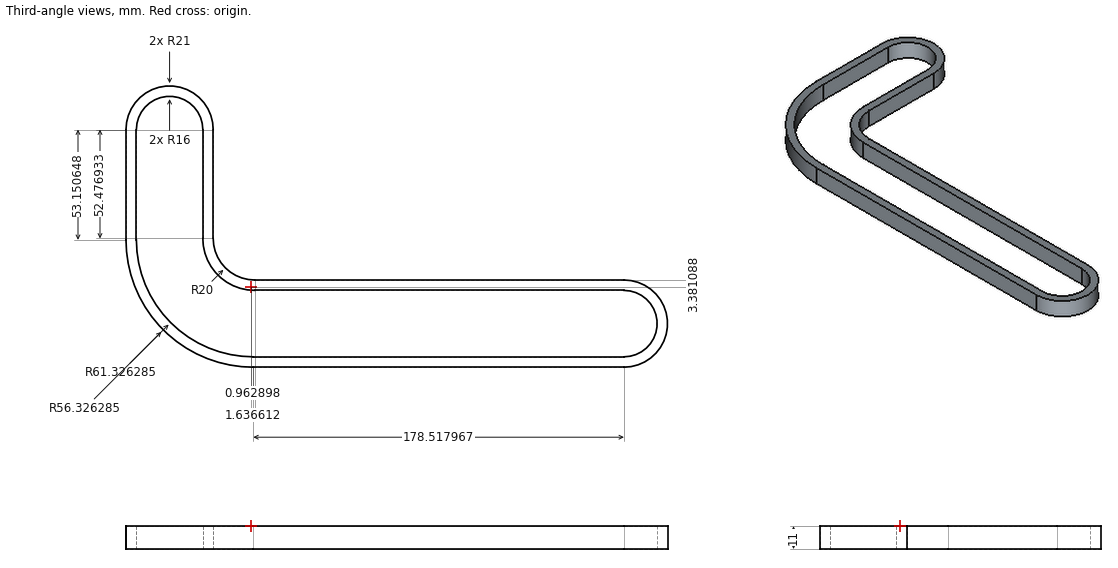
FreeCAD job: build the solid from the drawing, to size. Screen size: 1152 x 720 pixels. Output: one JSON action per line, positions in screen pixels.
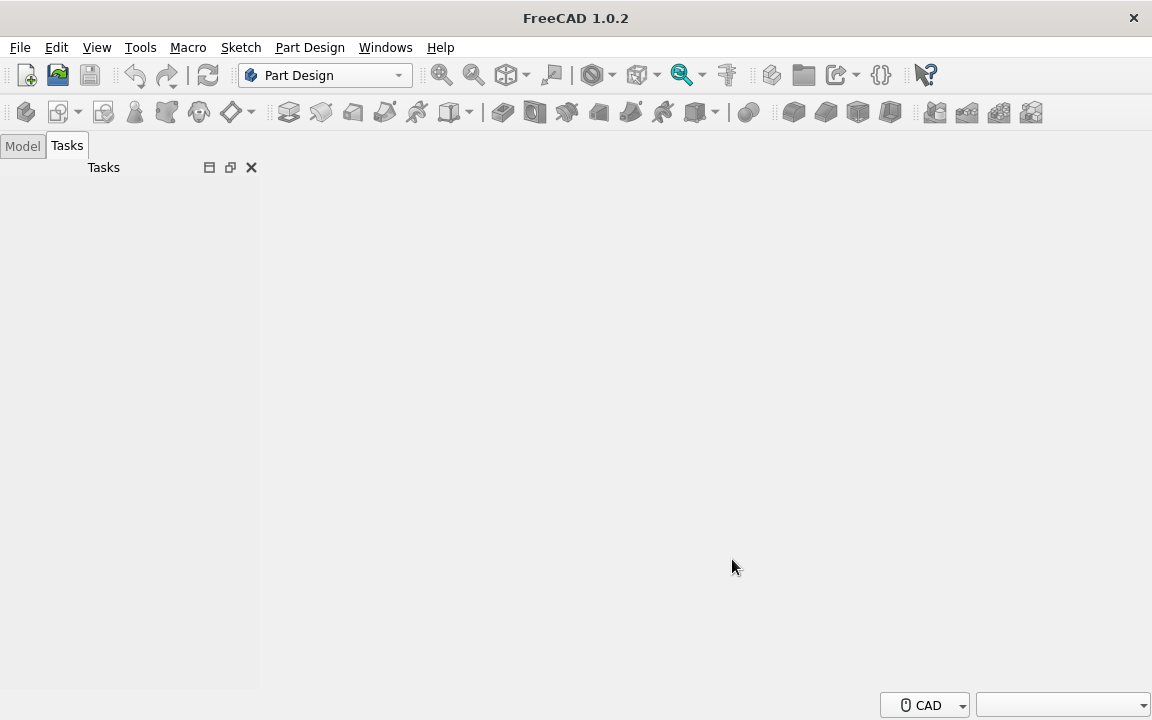
{"action": "key", "text": "ctrl+n"}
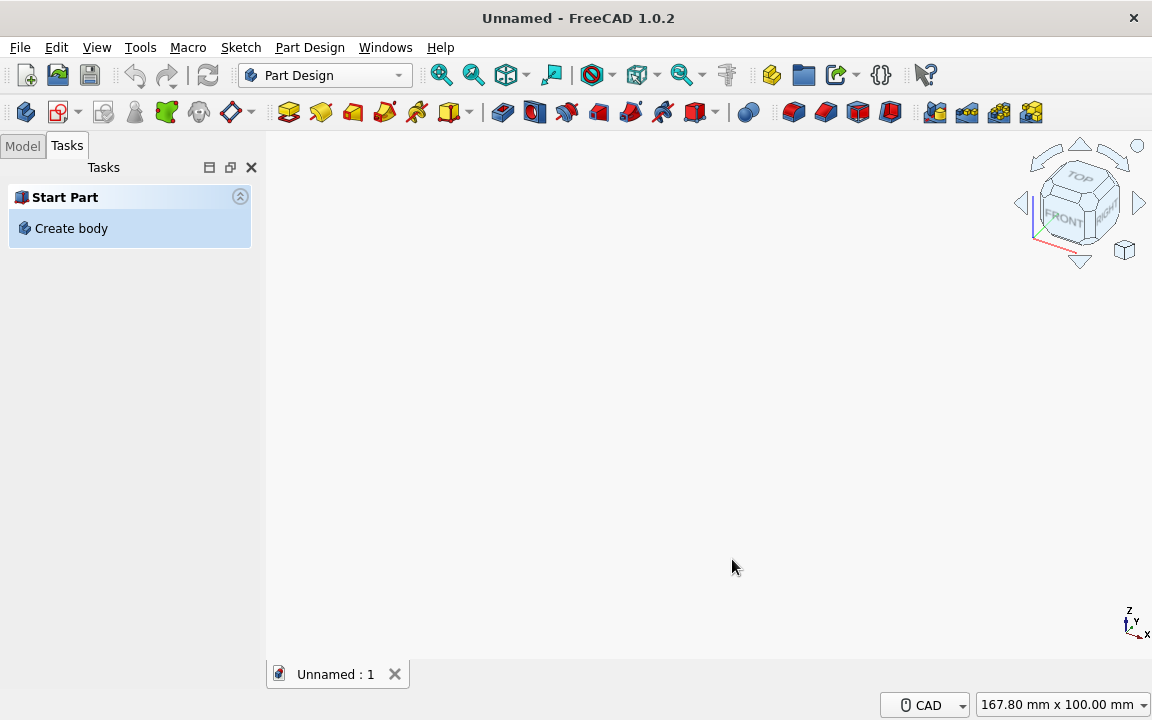
{"action": "left_click", "coordinate": [58, 112]}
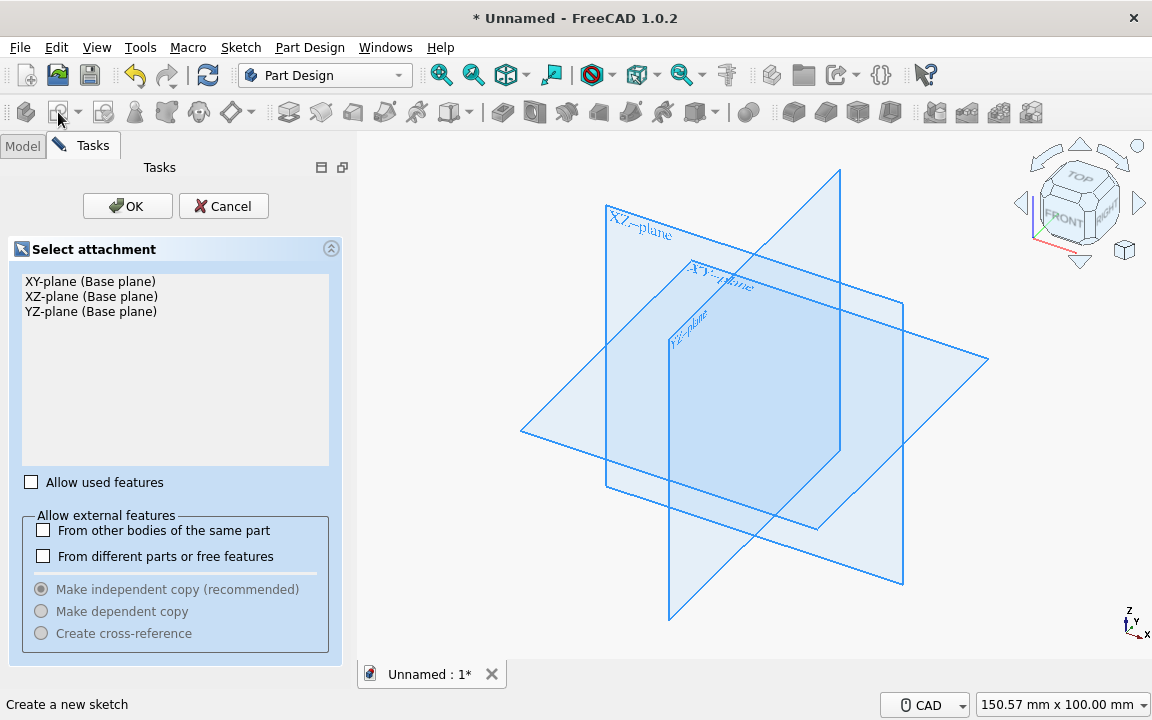
{"action": "left_click", "coordinate": [82, 282]}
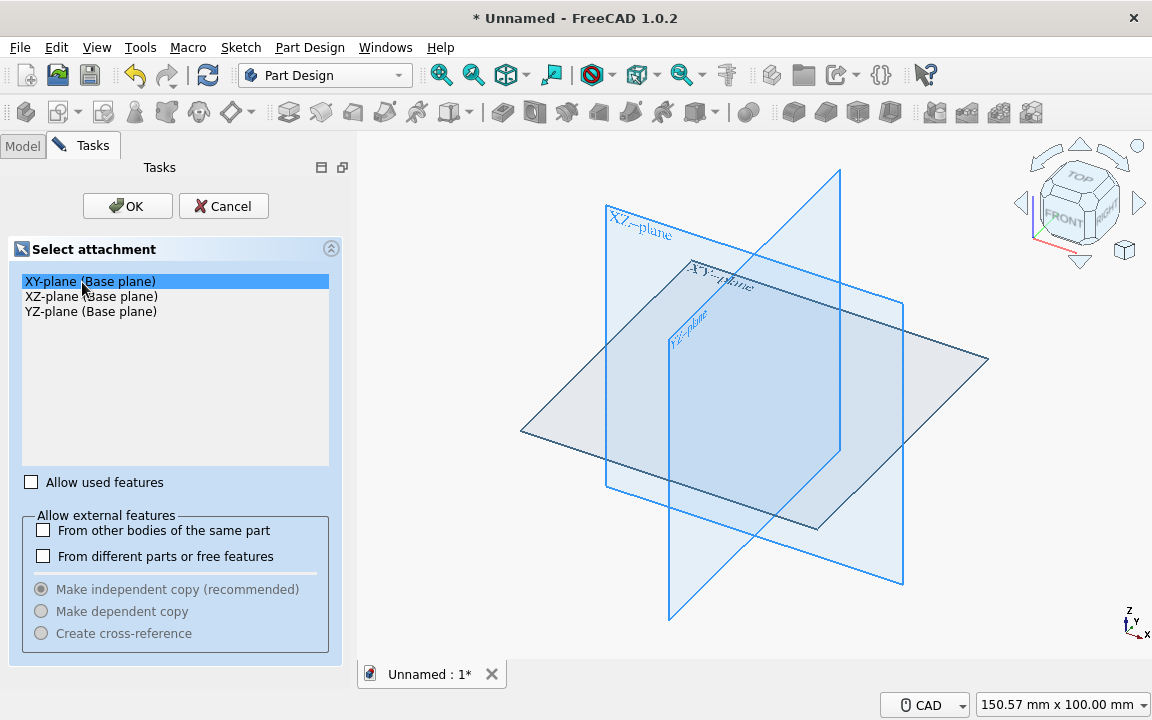
{"action": "left_click", "coordinate": [128, 206]}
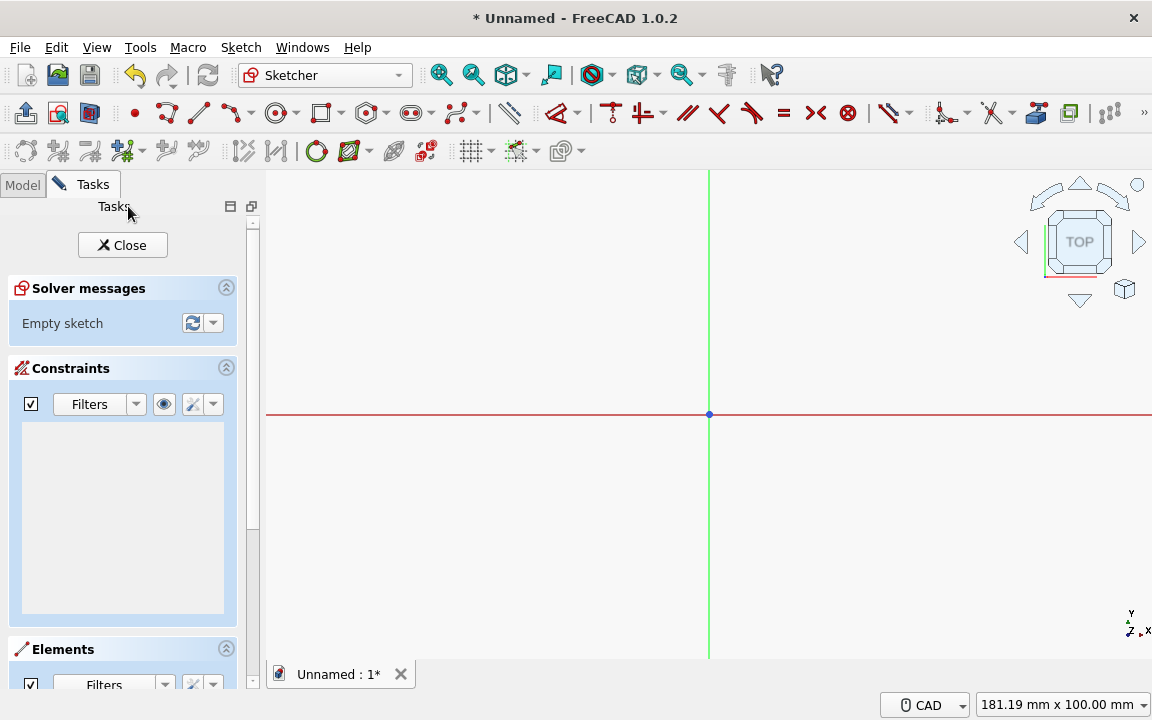
{"action": "scroll", "coordinate": [401, 497], "scroll_direction": "down", "scroll_amount": 5}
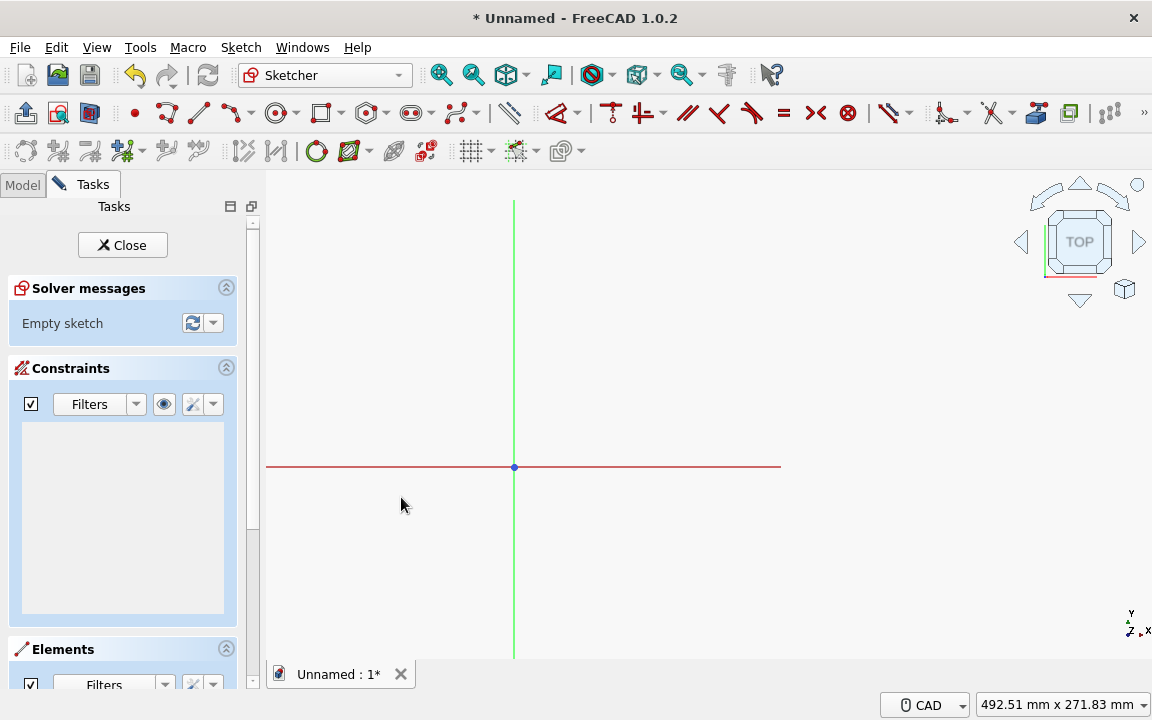
{"action": "left_click", "coordinate": [200, 114]}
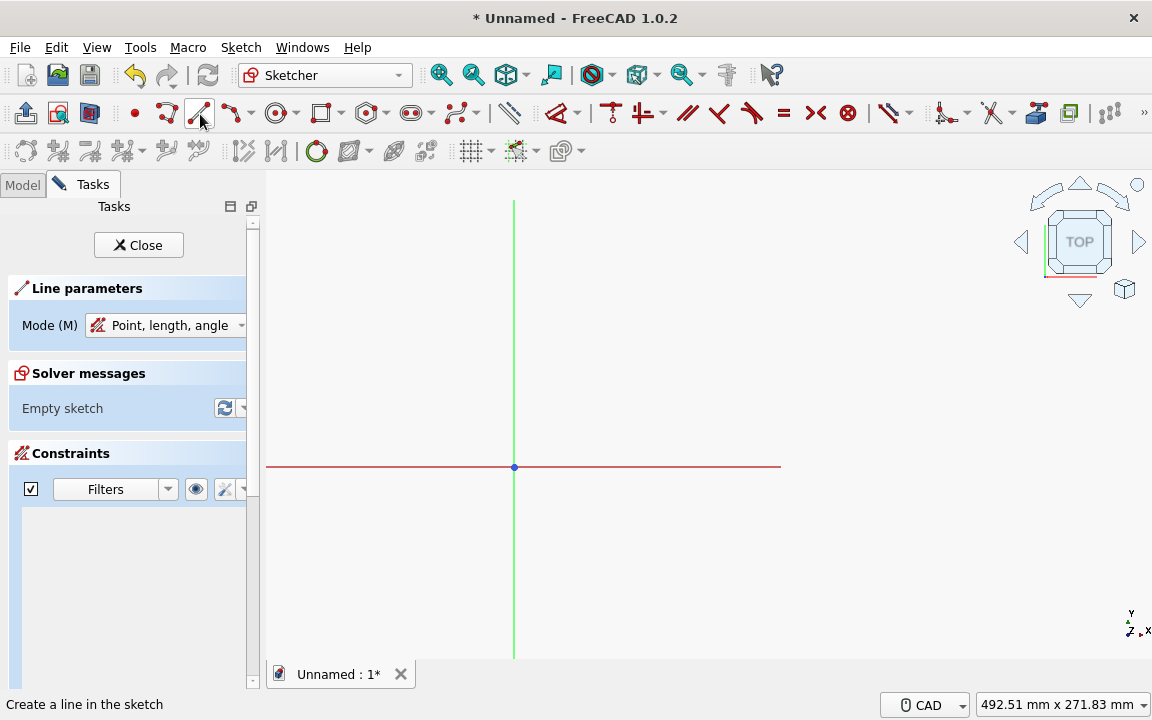
{"action": "left_click", "coordinate": [481, 425]}
{"action": "left_click", "coordinate": [481, 331]}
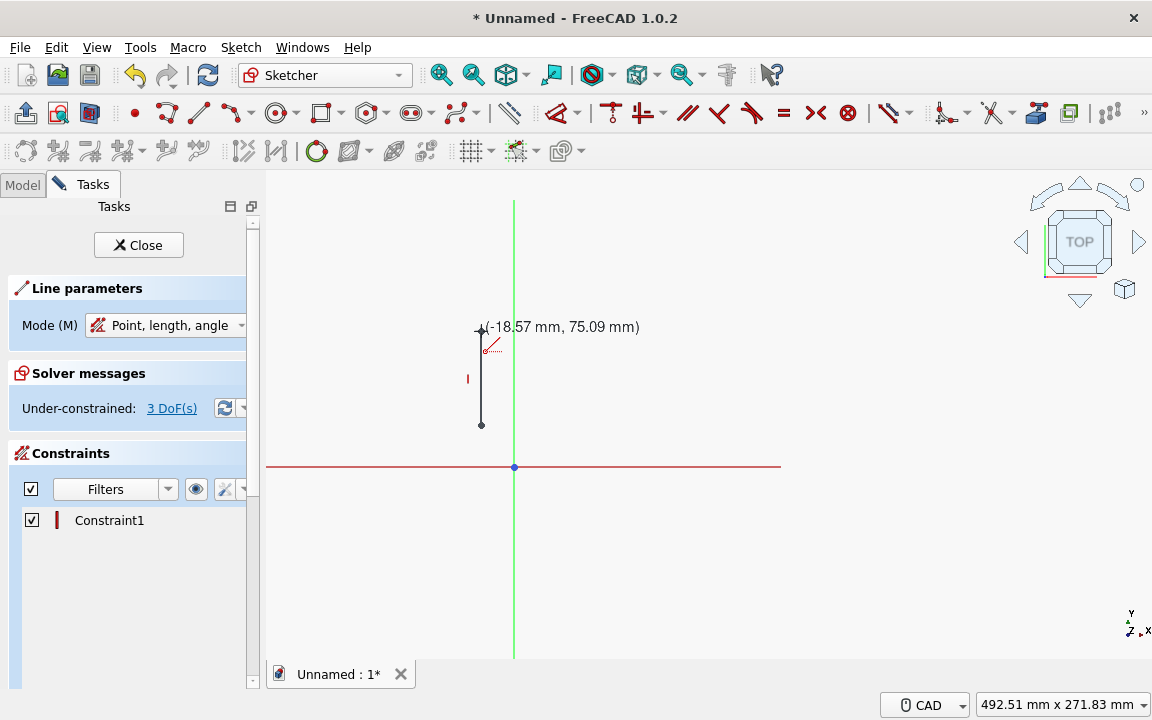
{"action": "left_click", "coordinate": [406, 331]}
{"action": "left_click", "coordinate": [406, 426]}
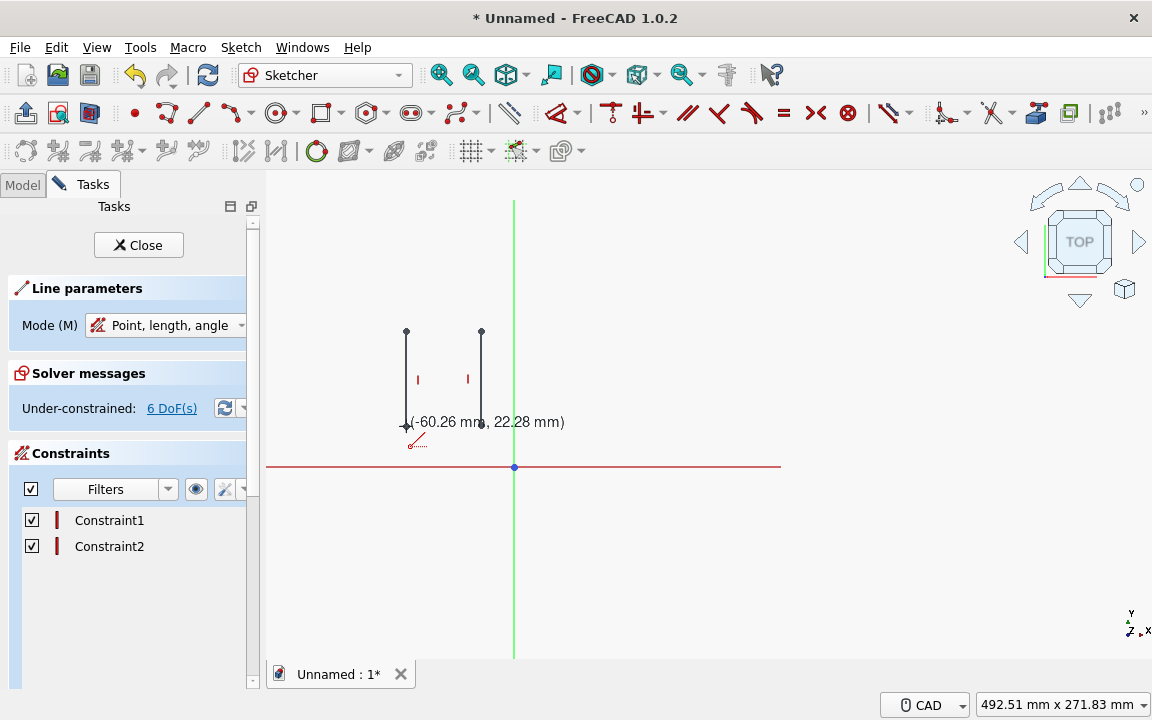
{"action": "scroll", "coordinate": [516, 537], "scroll_direction": "up", "scroll_amount": 12}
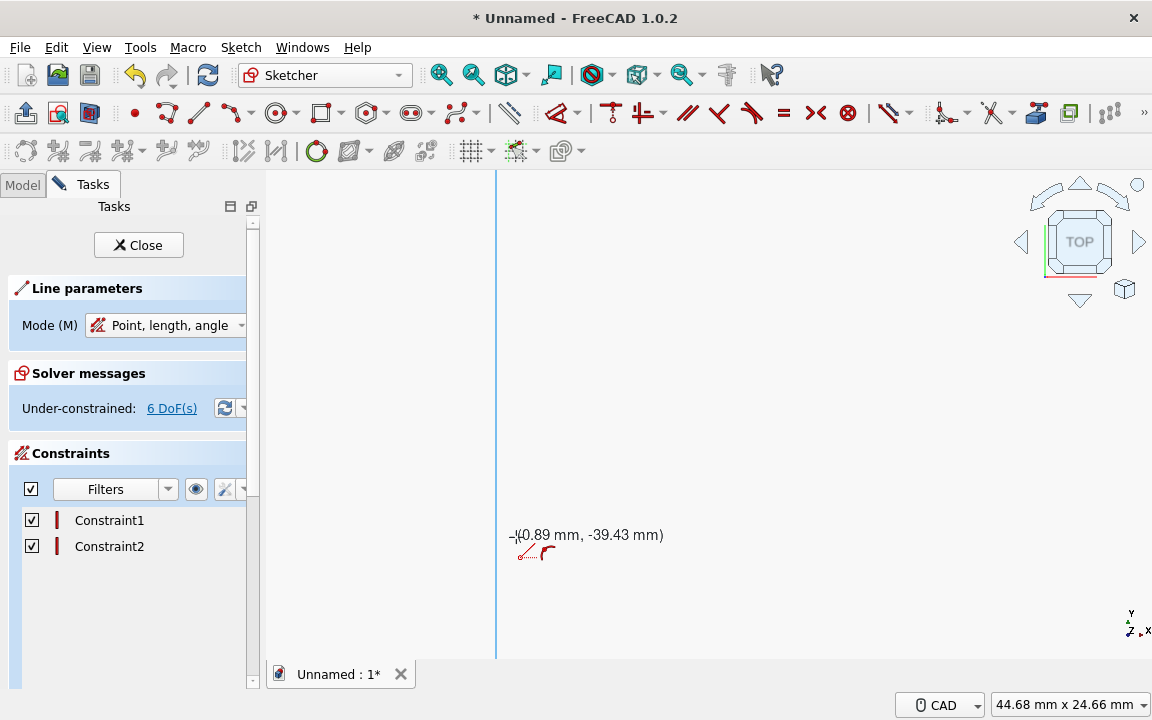
{"action": "left_click", "coordinate": [515, 524]}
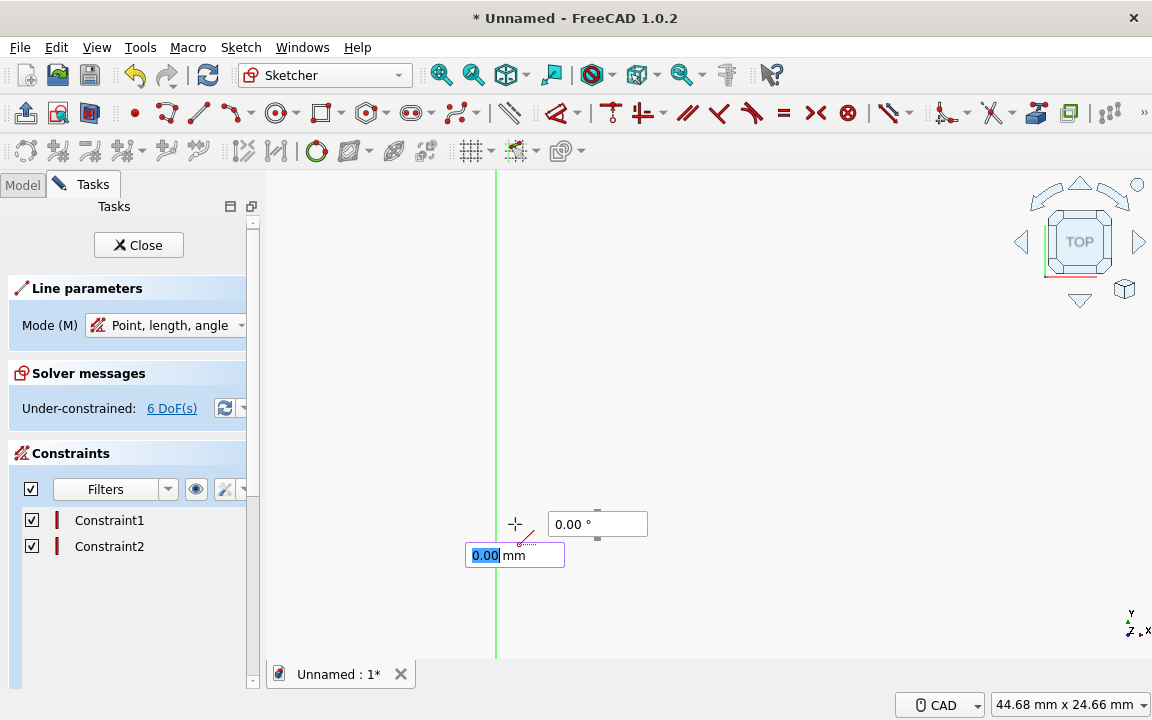
{"action": "scroll", "coordinate": [516, 538], "scroll_direction": "down", "scroll_amount": 12}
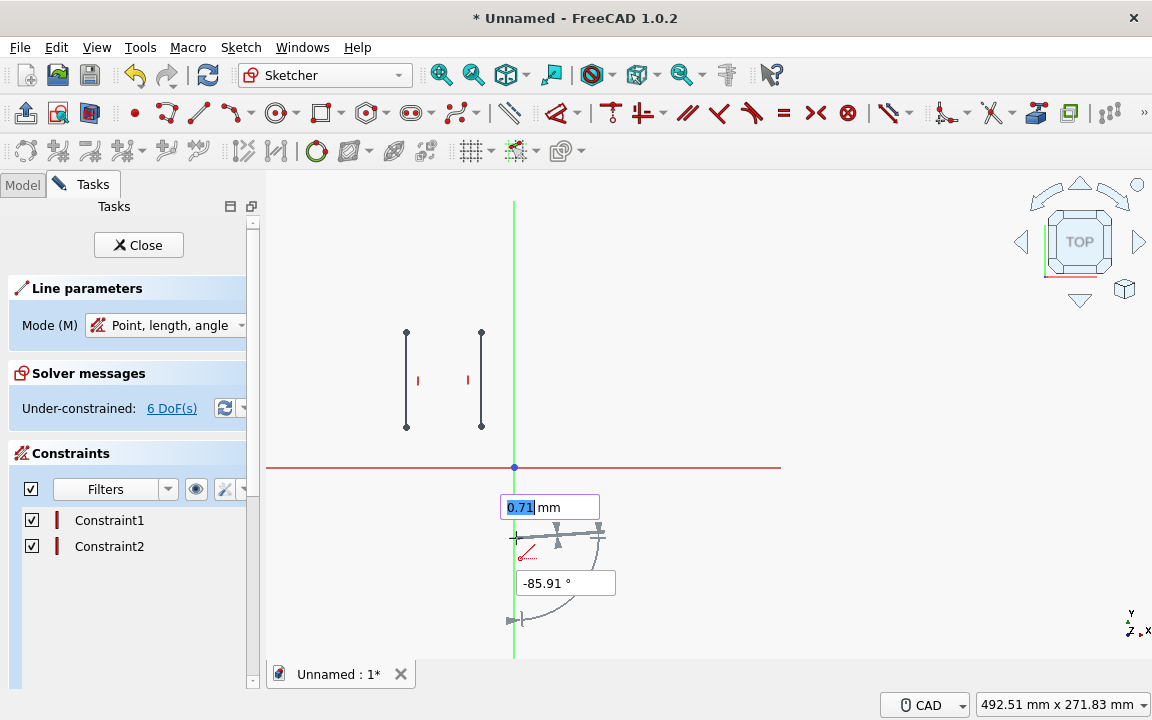
{"action": "left_click", "coordinate": [837, 537]}